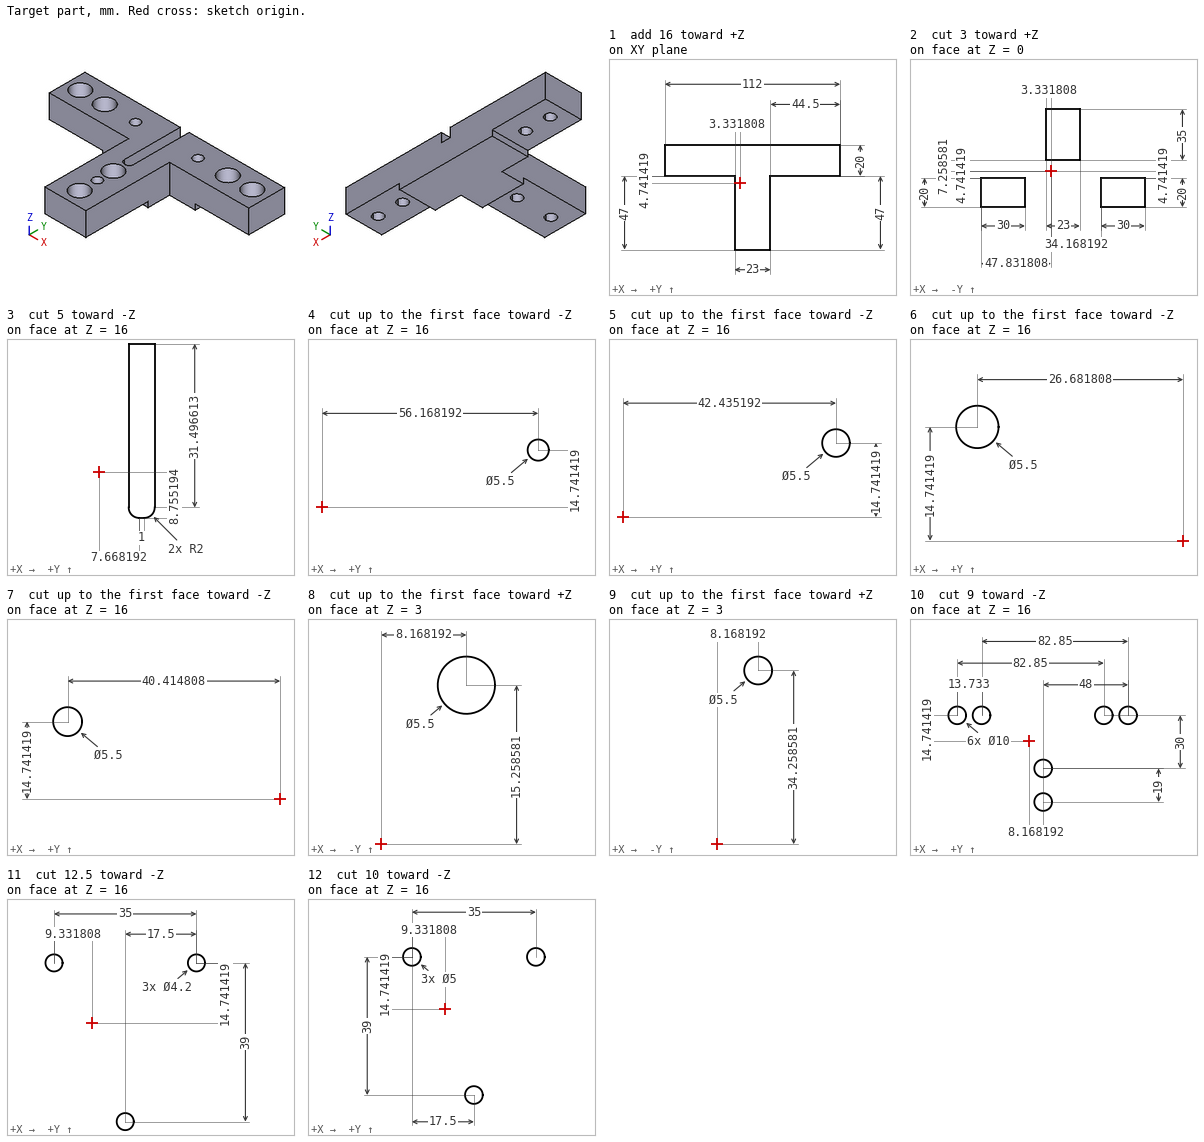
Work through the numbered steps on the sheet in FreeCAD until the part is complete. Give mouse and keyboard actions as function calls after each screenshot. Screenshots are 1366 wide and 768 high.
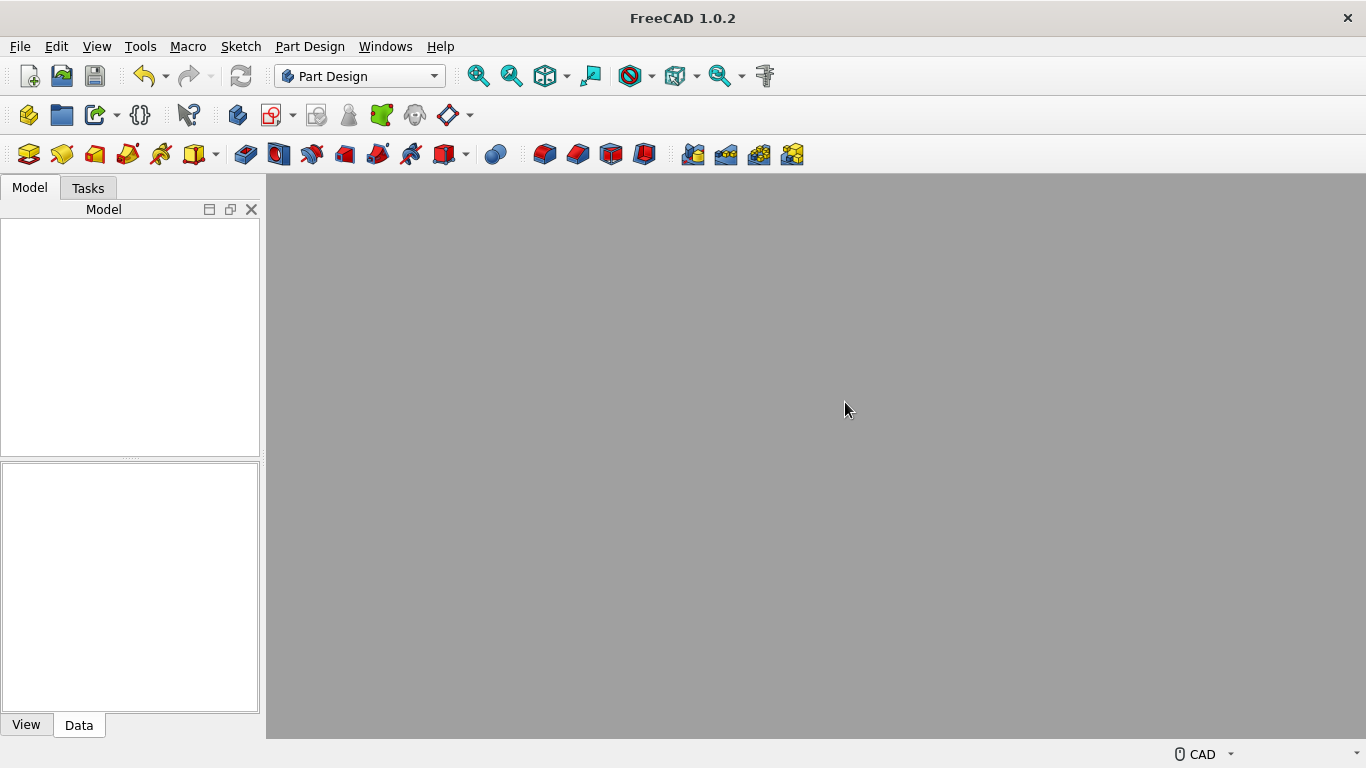
key(ctrl+n)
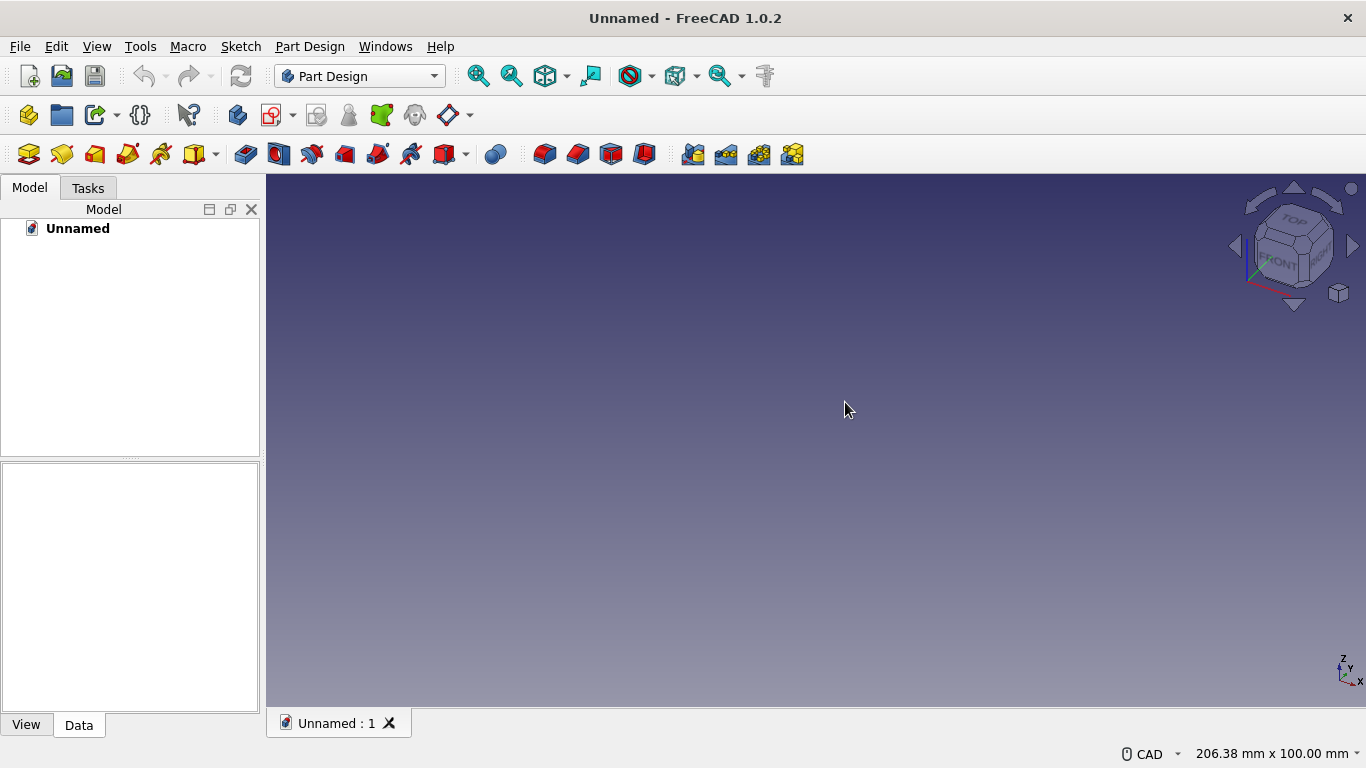
click(270, 116)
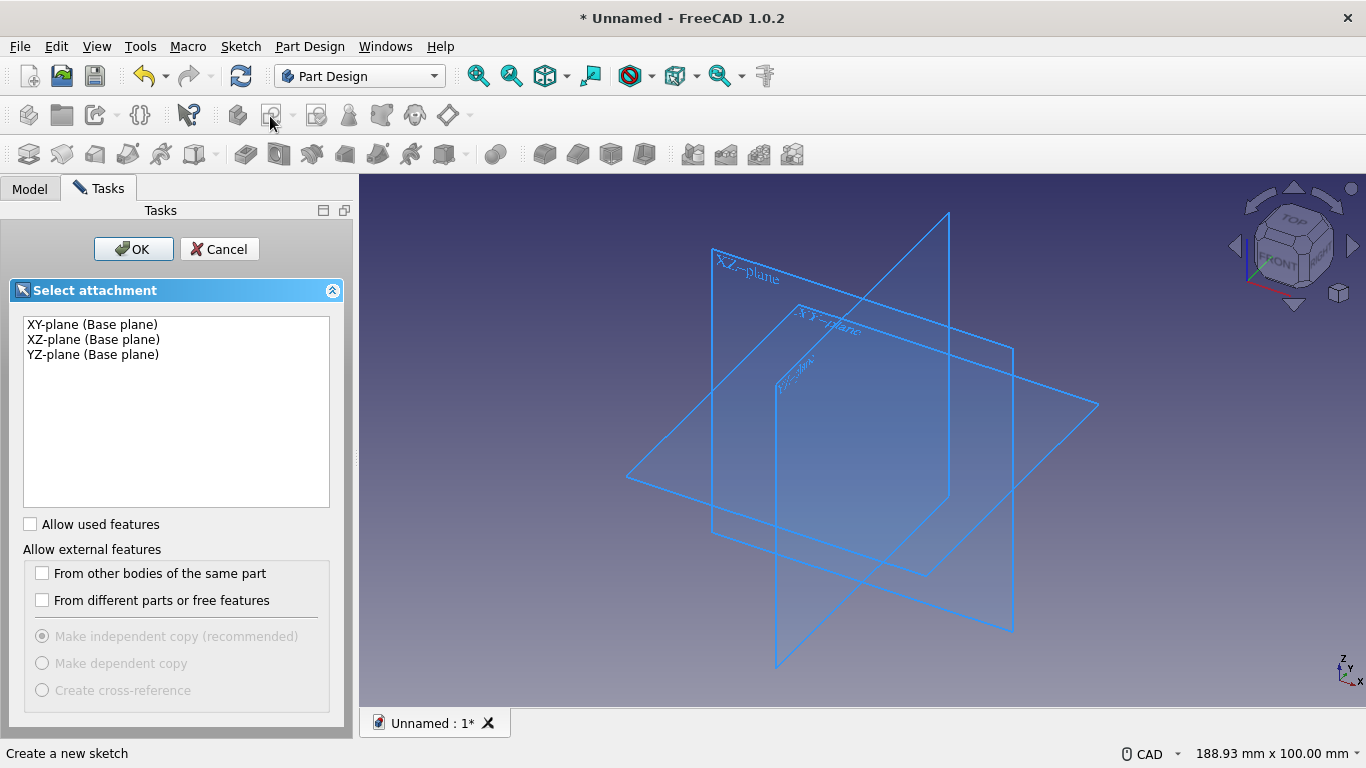
click(84, 324)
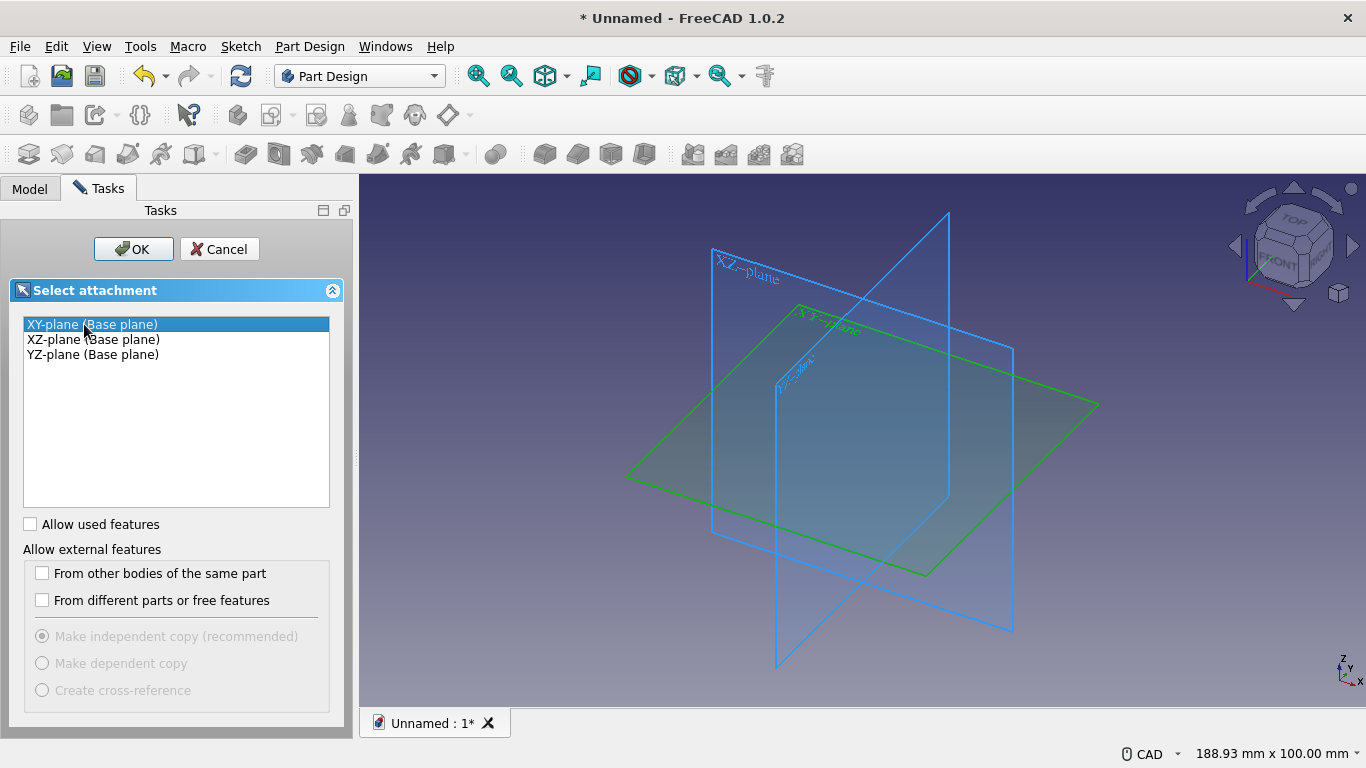
click(134, 249)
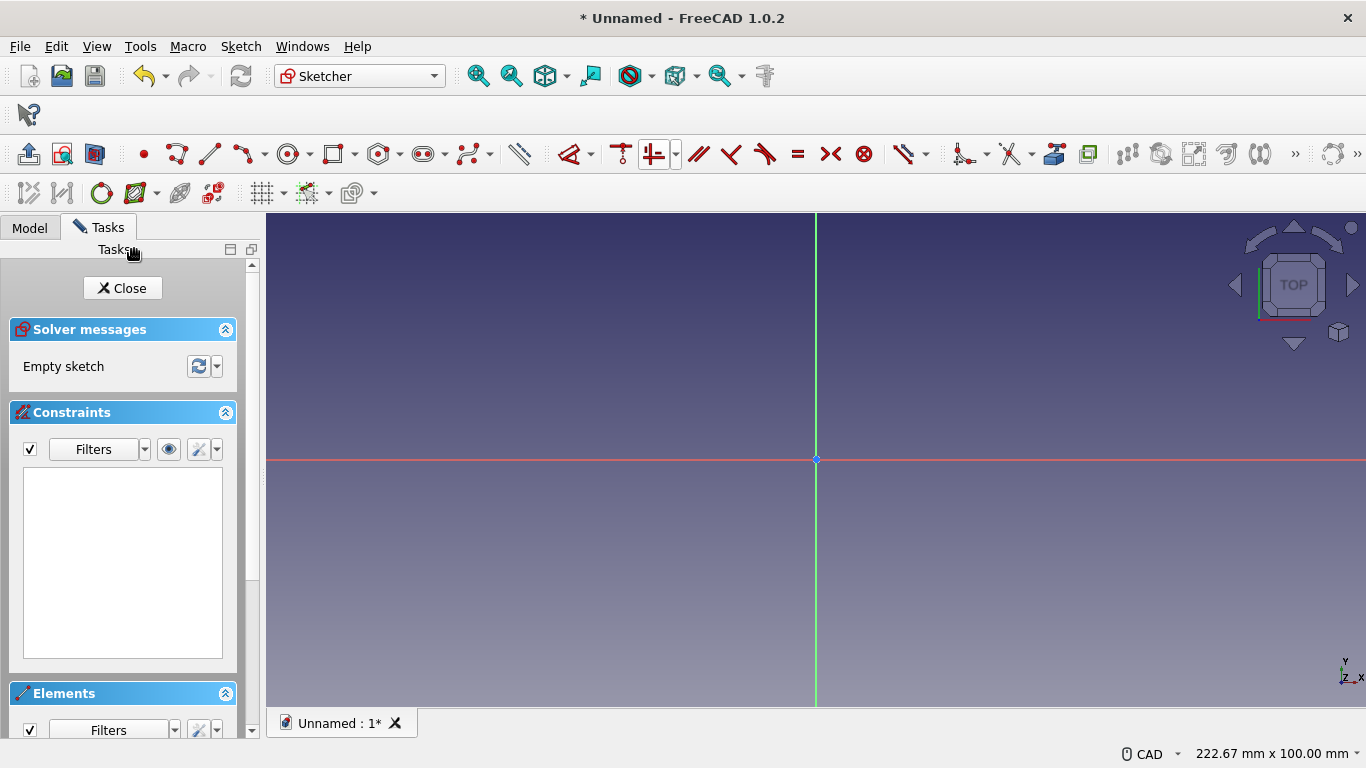
scroll(294, 265, down, 1)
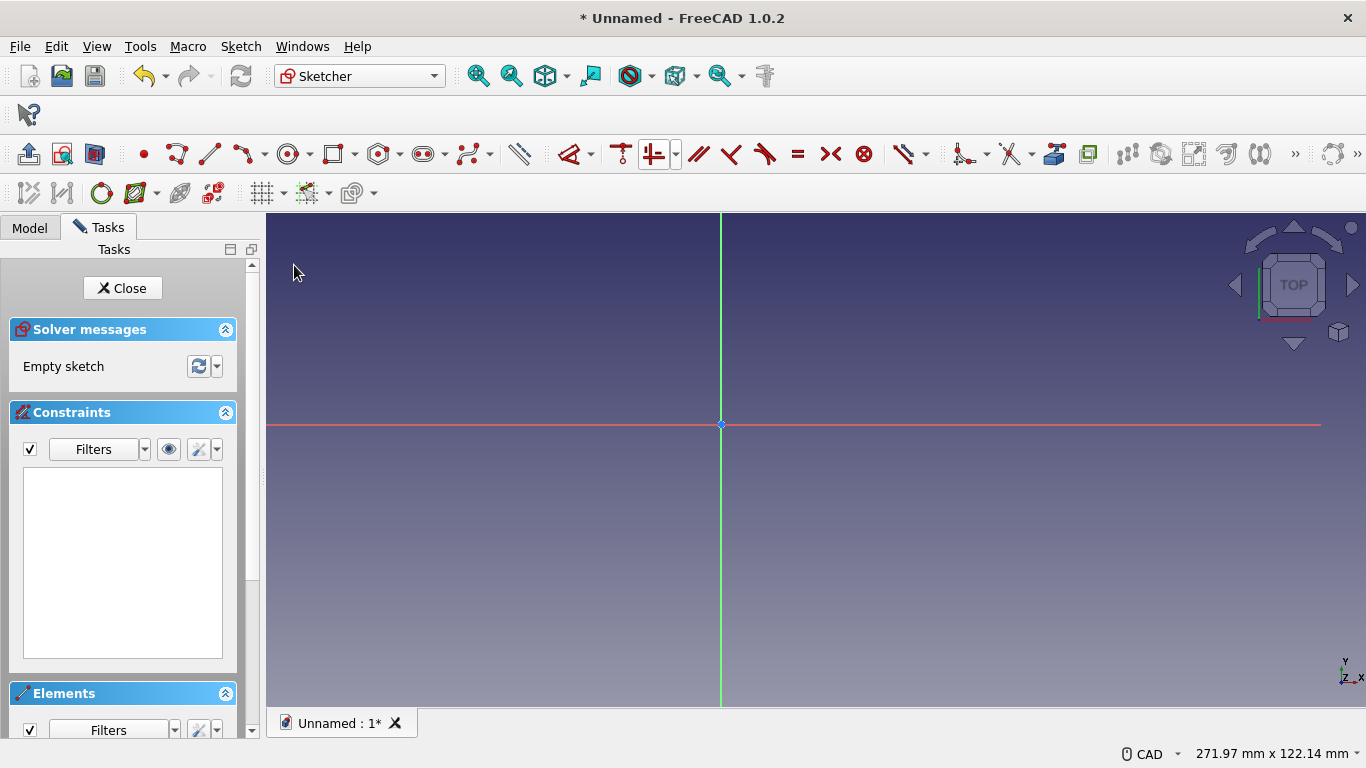
click(177, 154)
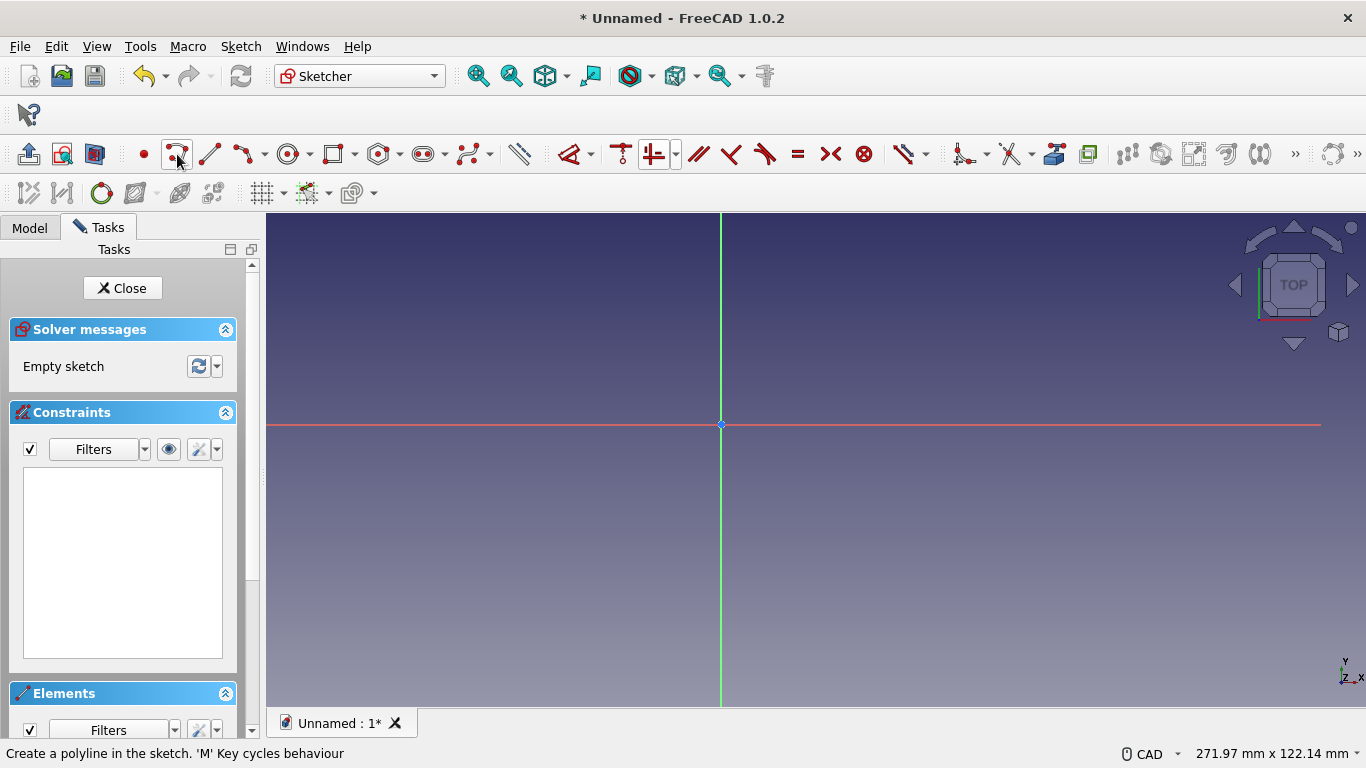
click(708, 405)
click(708, 596)
click(801, 596)
click(801, 405)
click(981, 405)
click(981, 325)
click(528, 325)
click(528, 405)
click(708, 406)
key(Escape)
key(Escape)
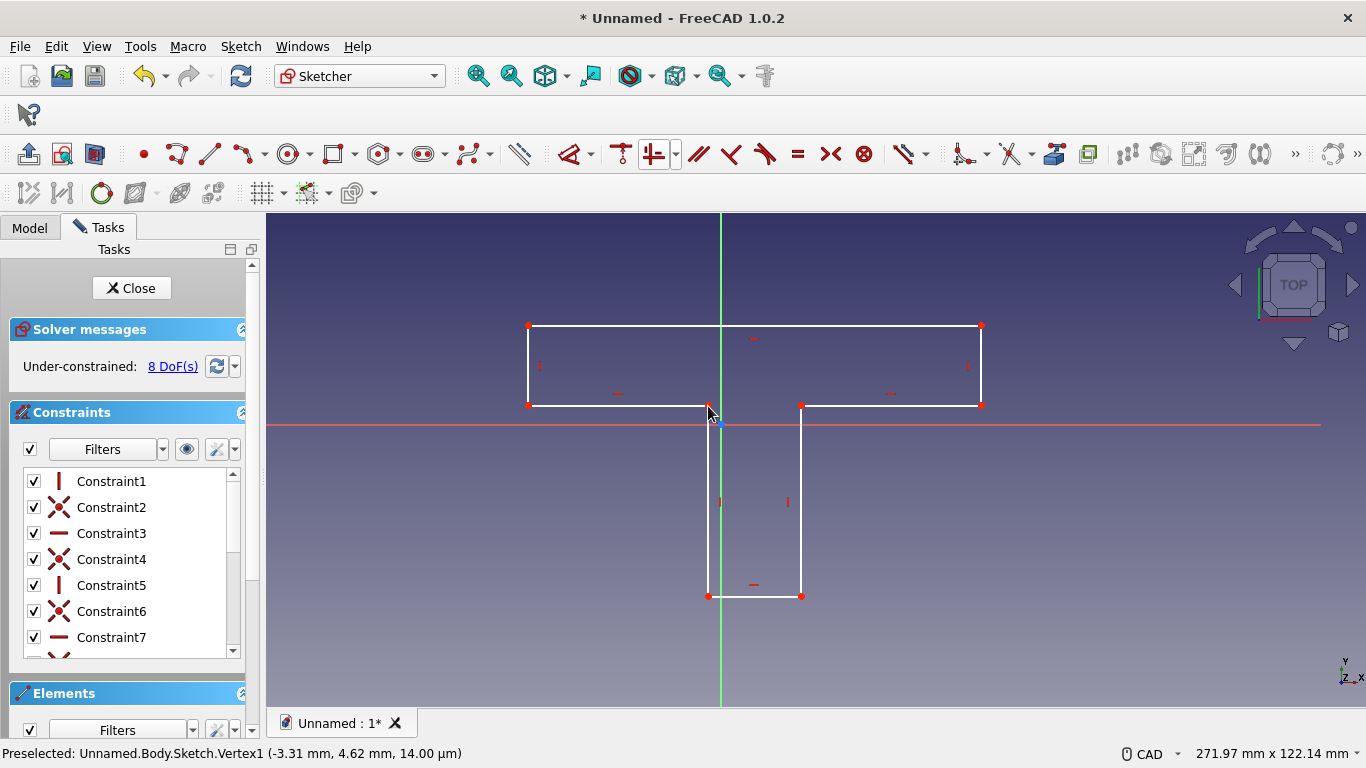
click(568, 154)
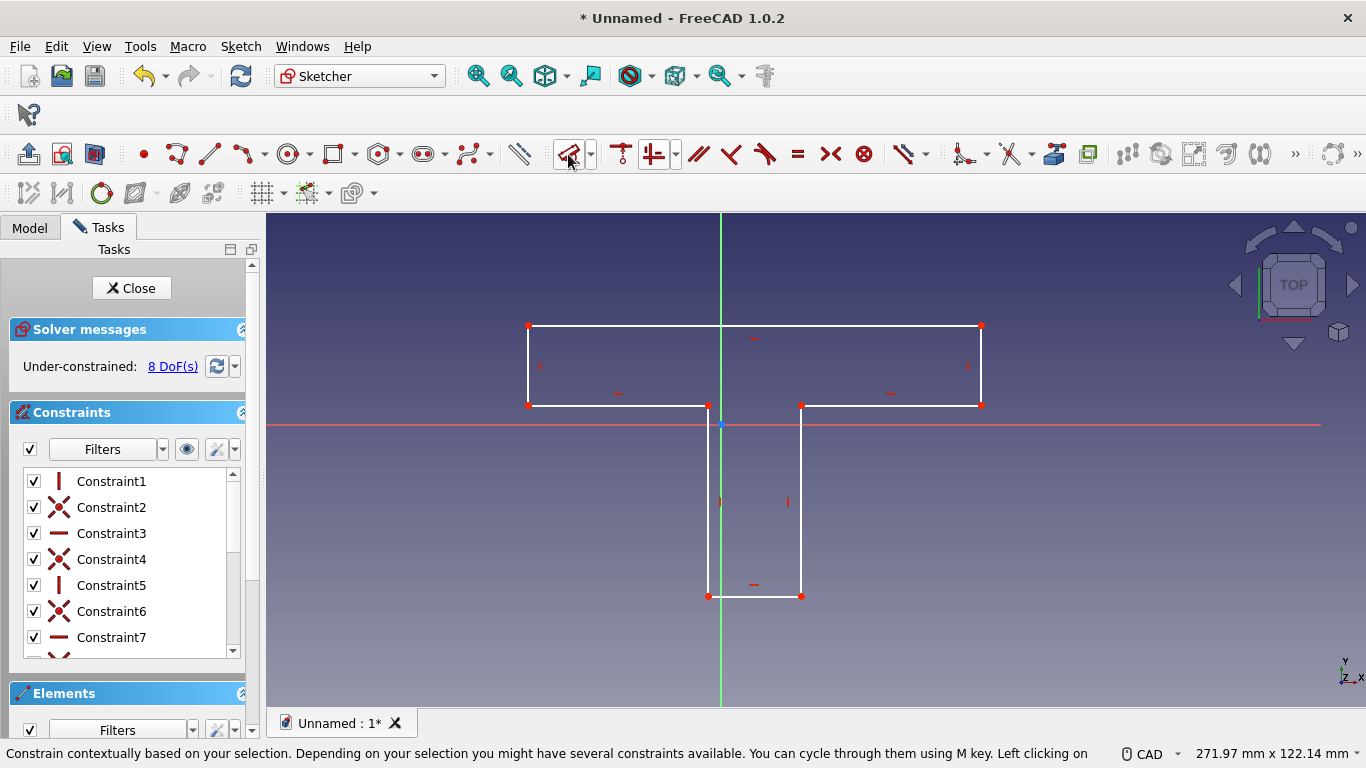
click(708, 463)
click(674, 501)